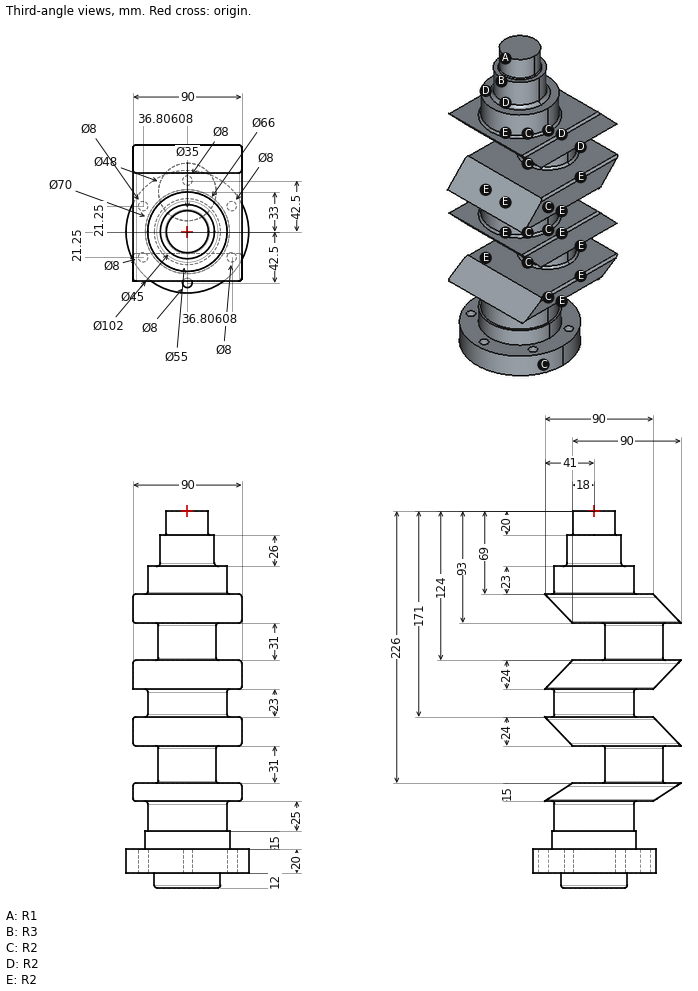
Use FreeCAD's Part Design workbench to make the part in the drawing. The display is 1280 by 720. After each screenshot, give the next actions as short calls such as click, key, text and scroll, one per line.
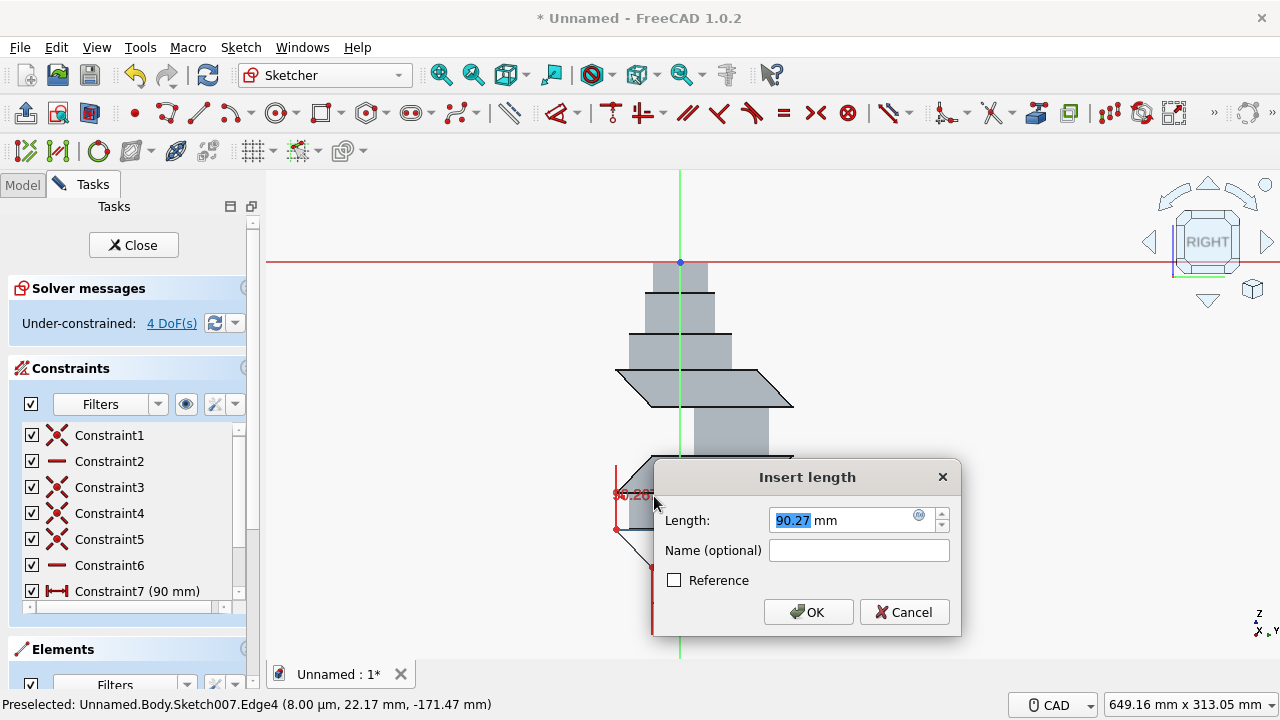
text(90)
key(Return)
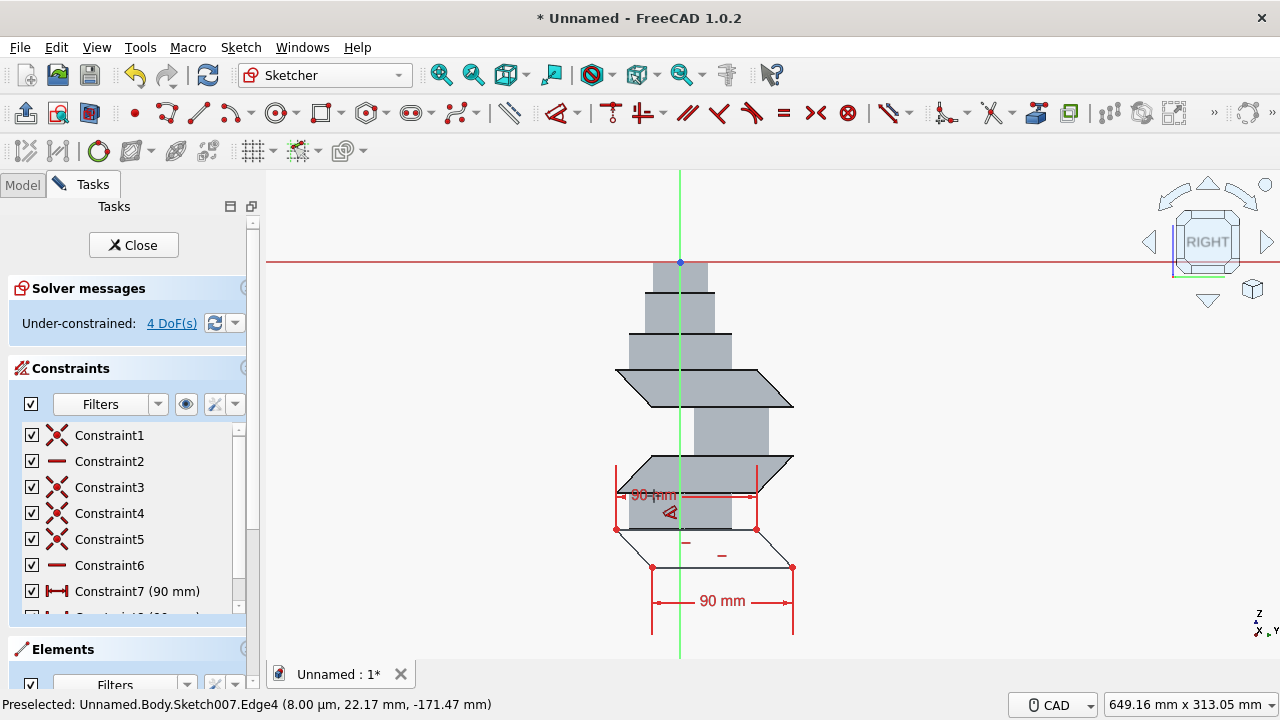
click(616, 530)
click(648, 228)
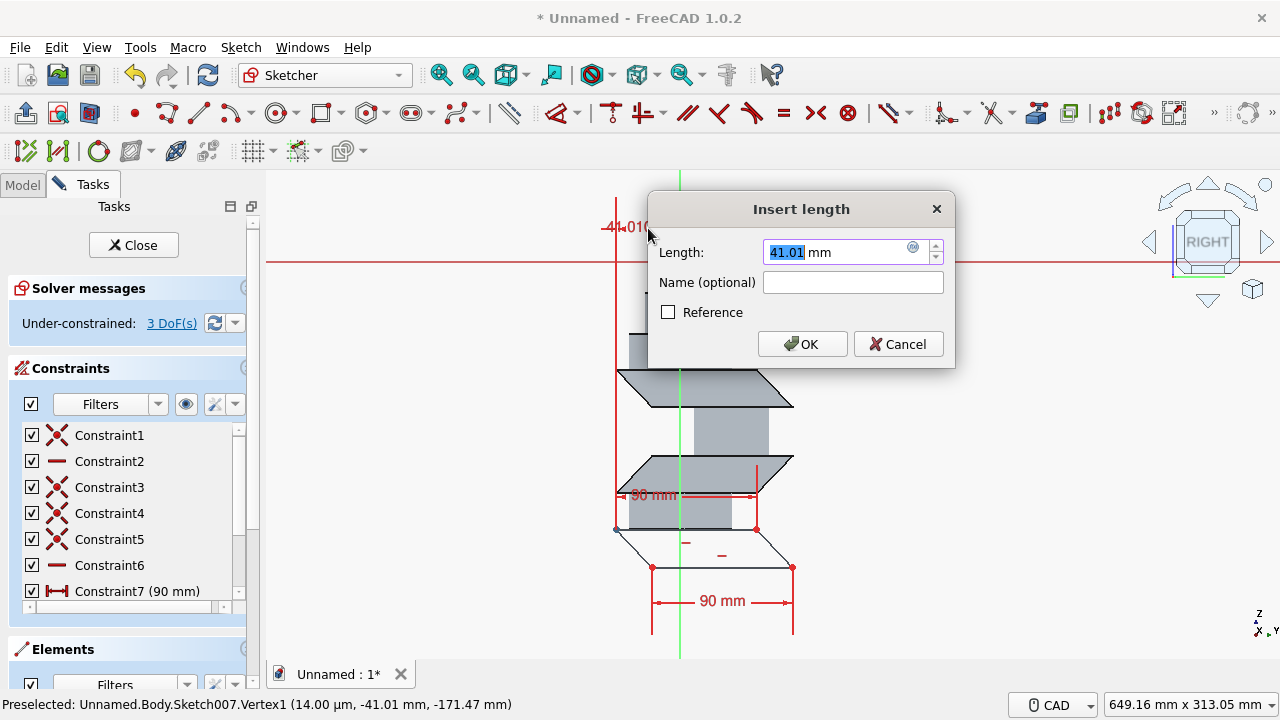
text(41)
key(Return)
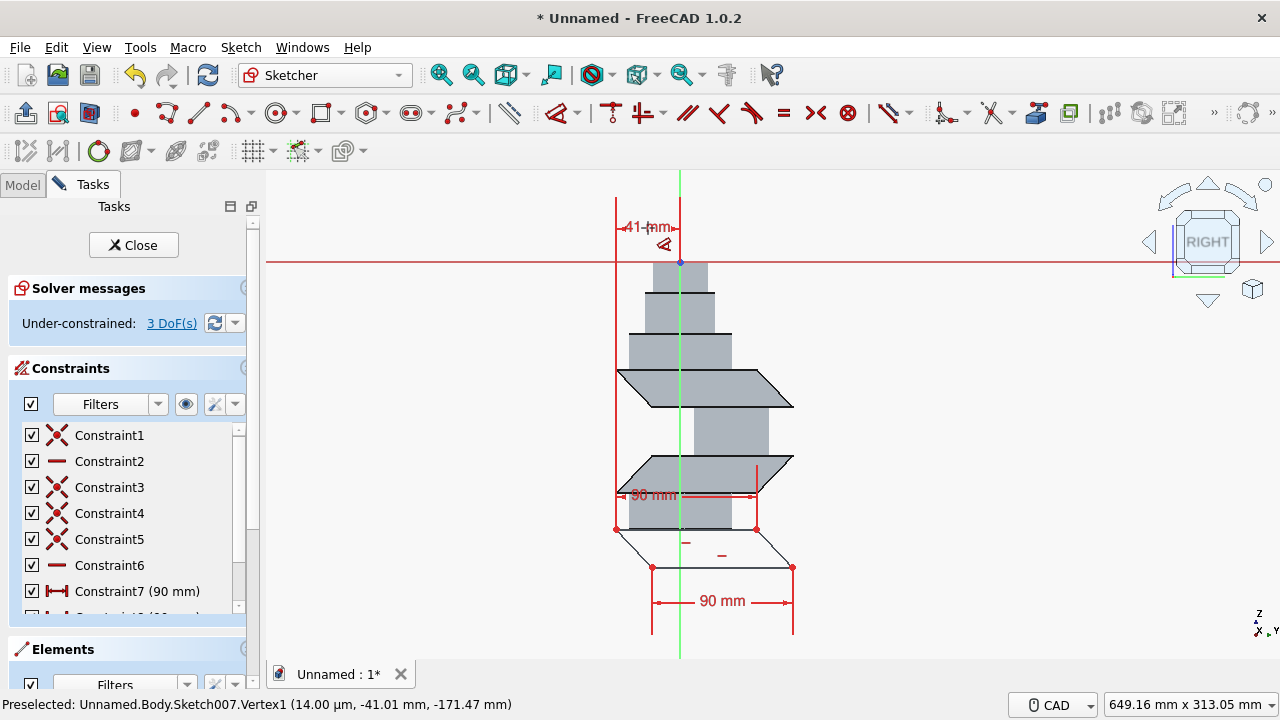
scroll(652, 568, up, 2)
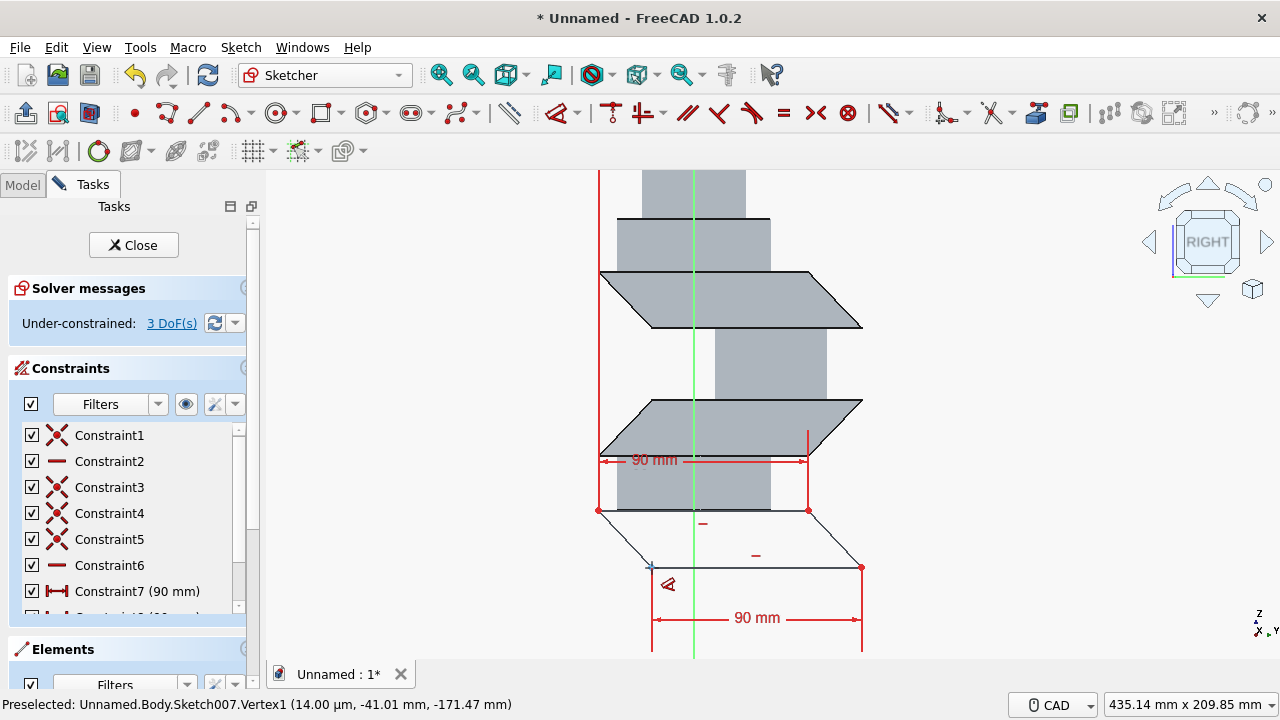
click(652, 568)
click(673, 602)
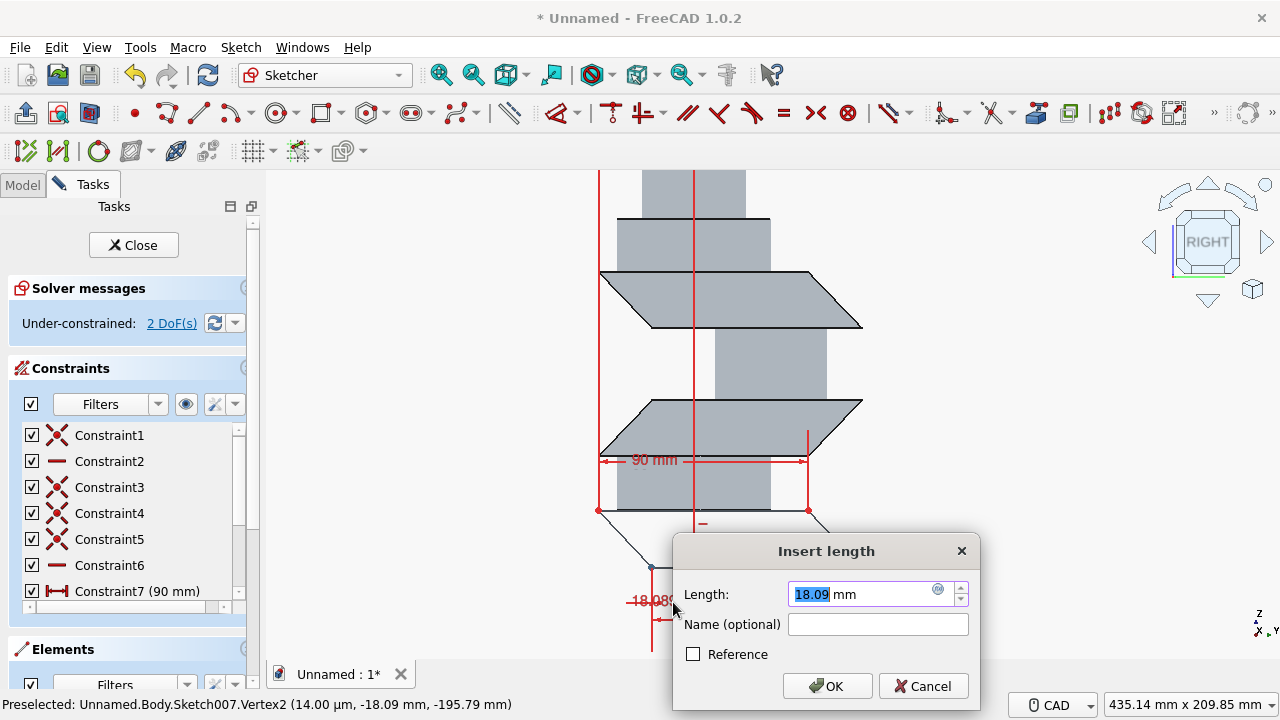
text(18)
key(Return)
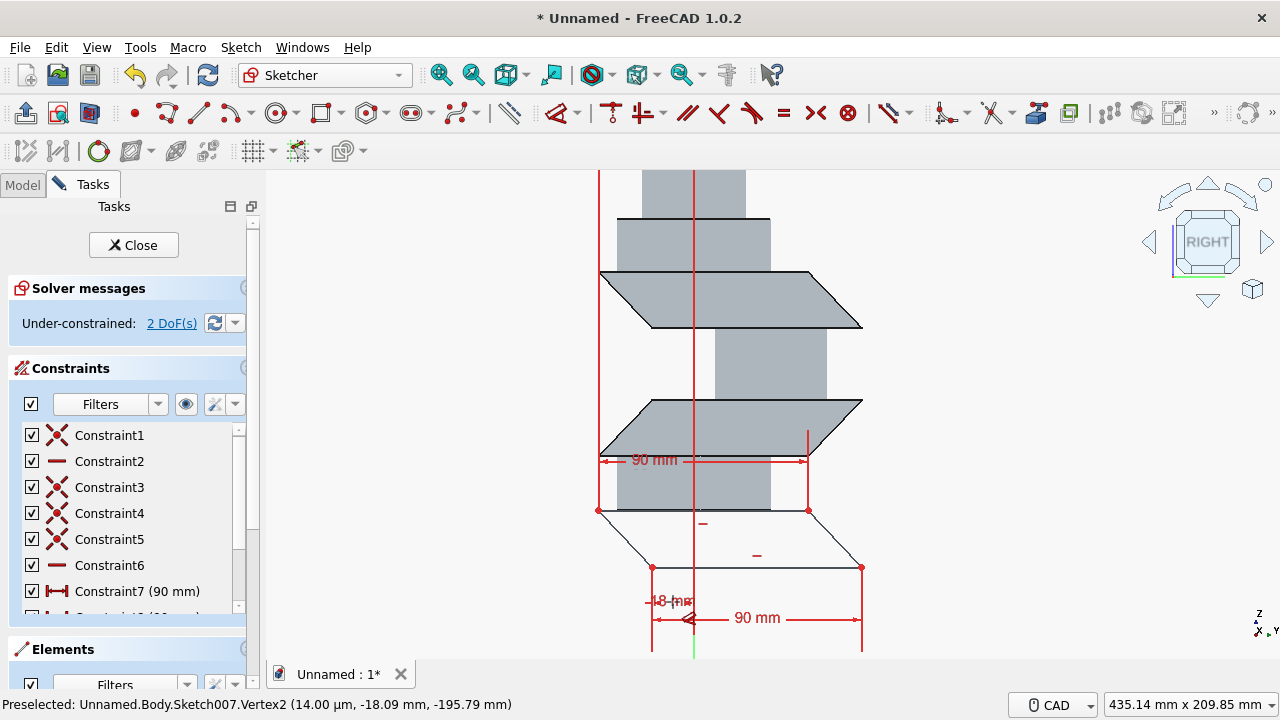
click(615, 528)
click(565, 539)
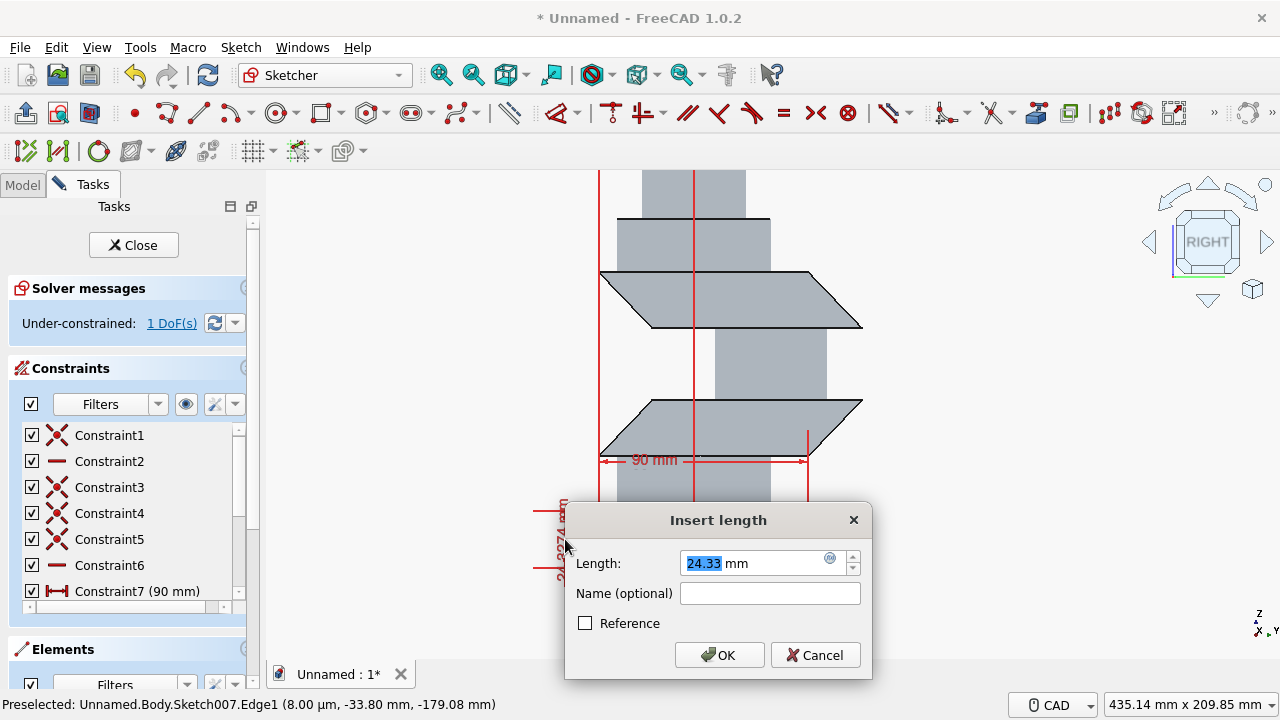
text(24)
key(Return)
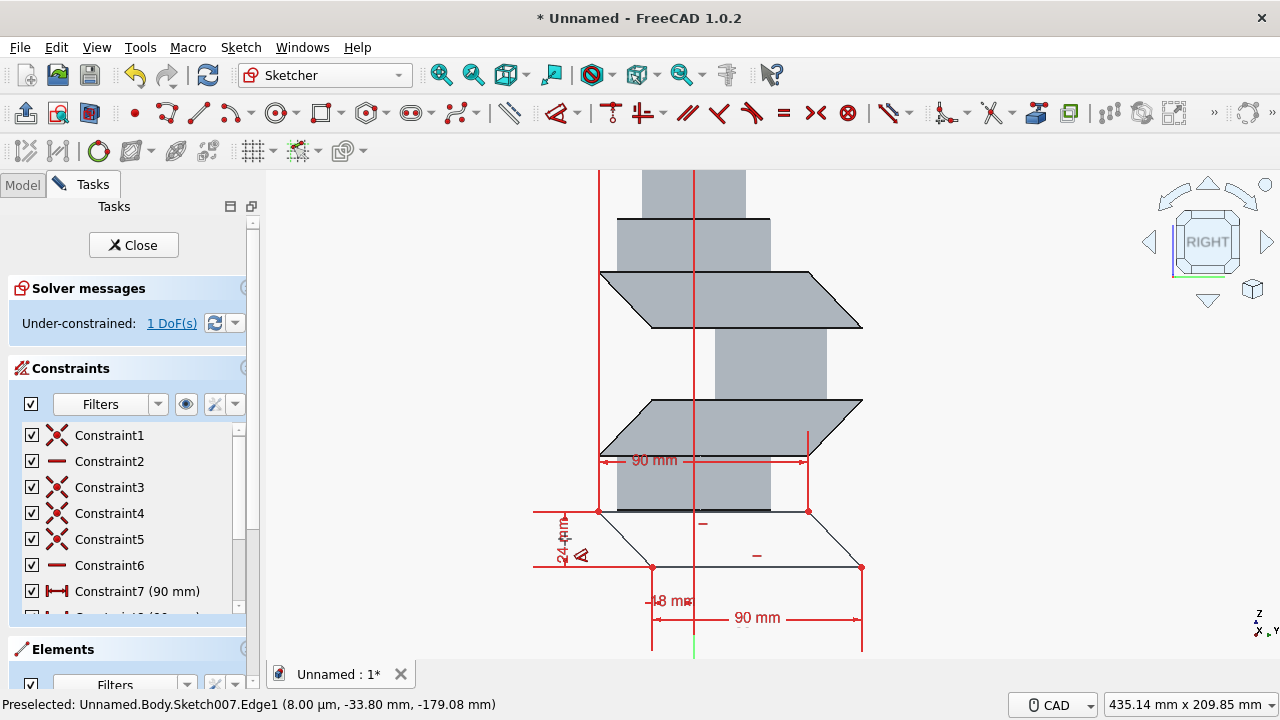
click(599, 512)
click(565, 355)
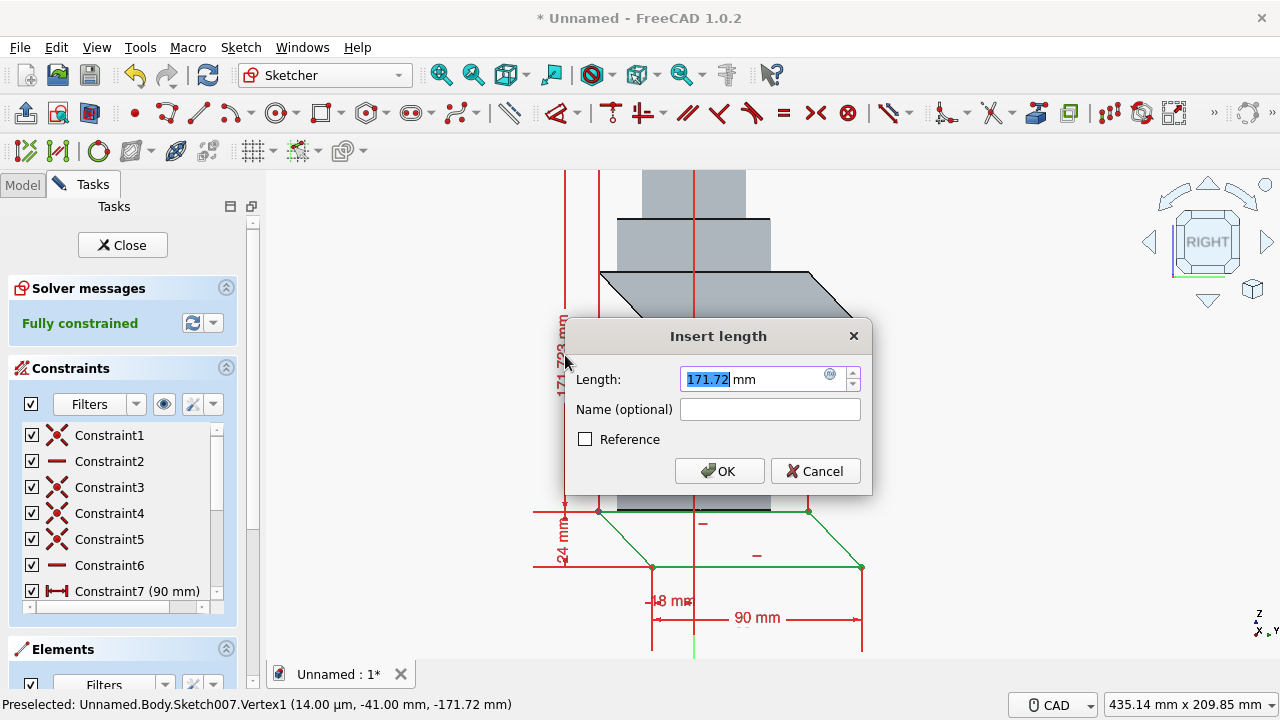
text(171)
key(Return)
key(Escape)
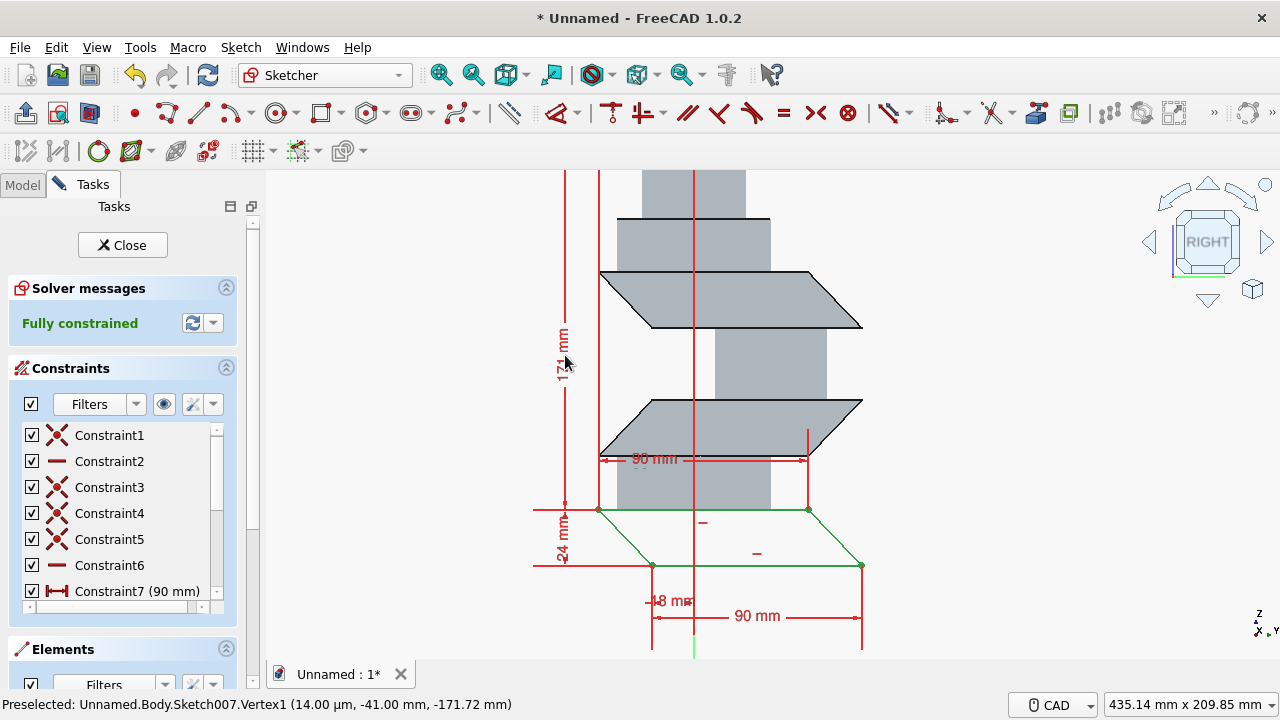
click(123, 245)